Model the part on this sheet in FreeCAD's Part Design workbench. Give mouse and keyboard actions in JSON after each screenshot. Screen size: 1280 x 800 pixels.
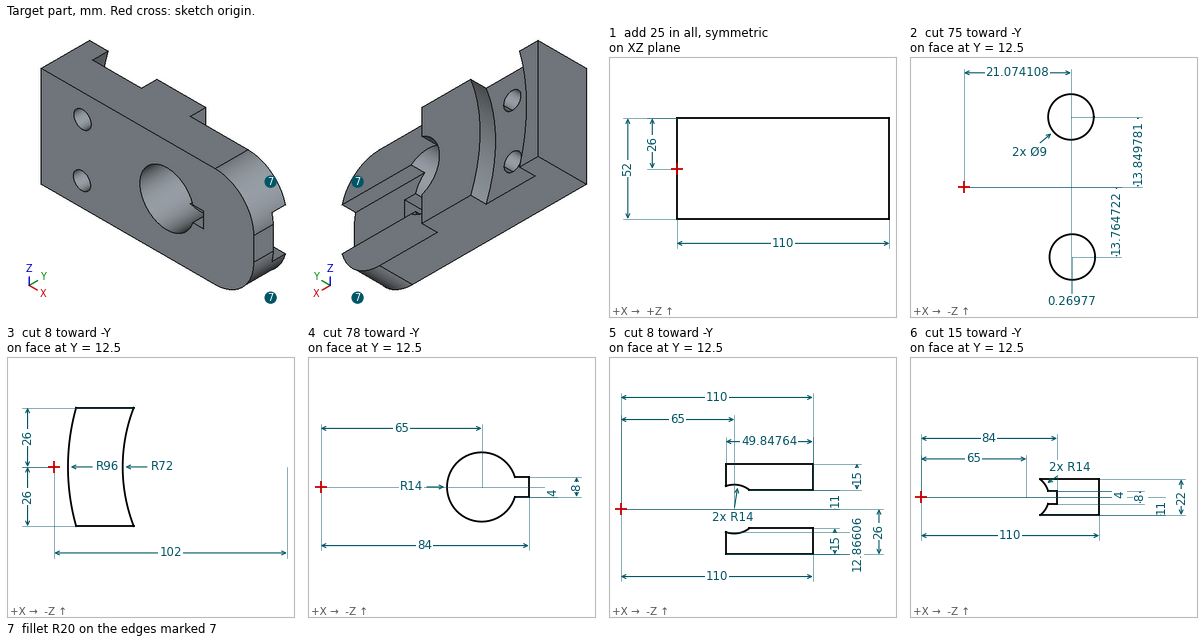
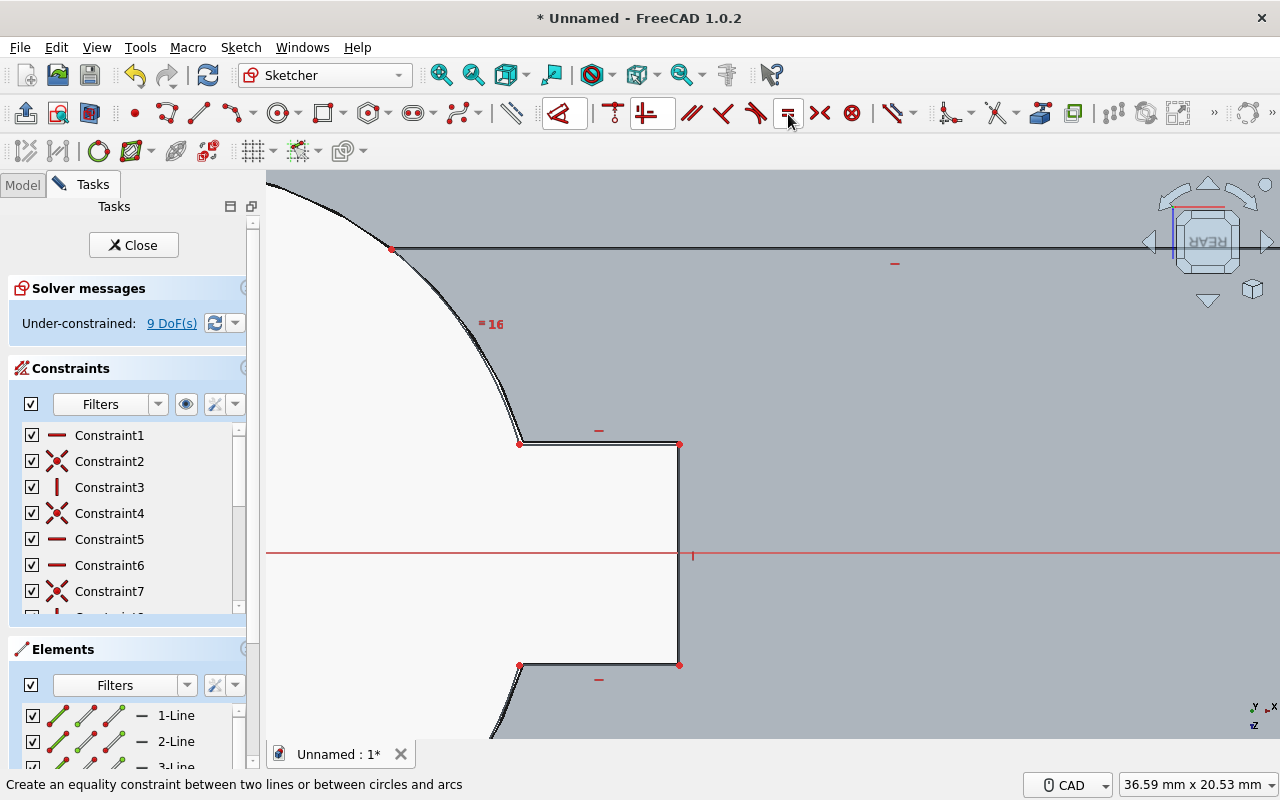
{"action": "scroll", "coordinate": [472, 334], "scroll_direction": "down", "scroll_amount": 3}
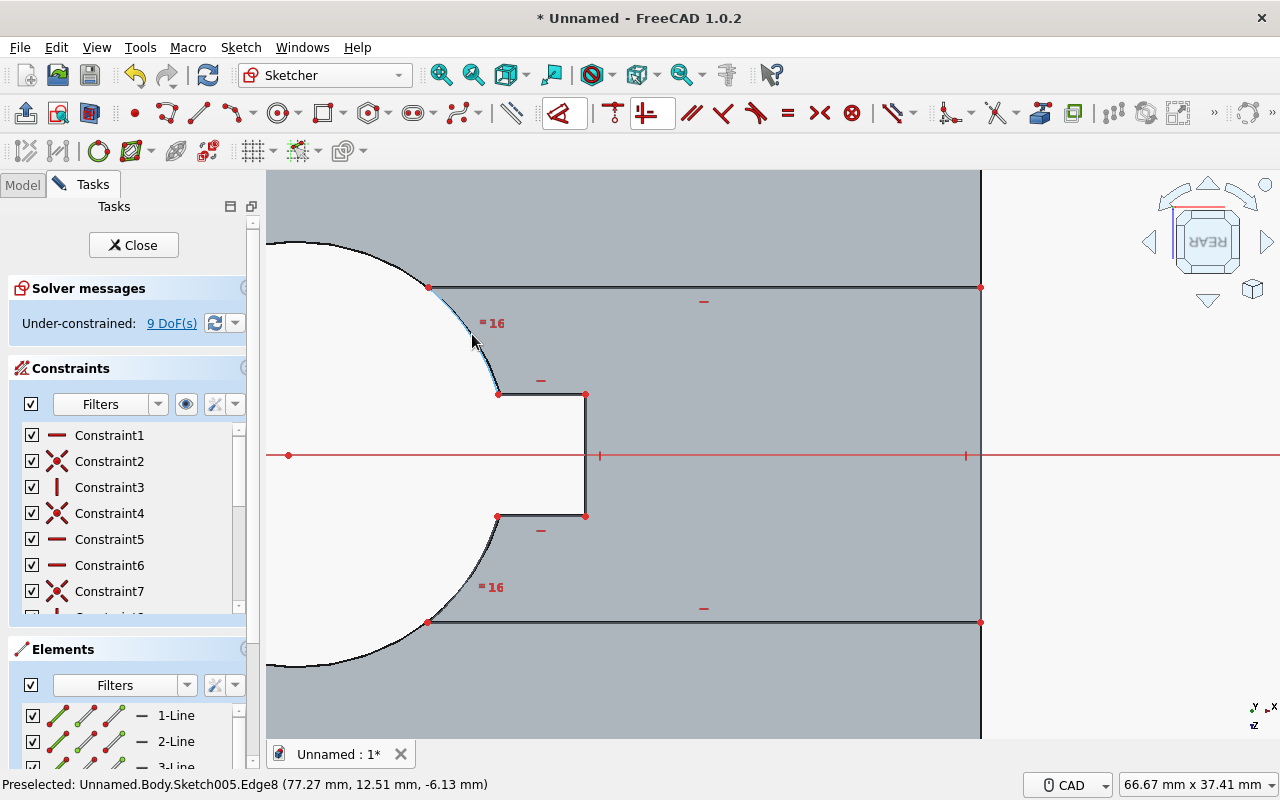
{"action": "scroll", "coordinate": [1020, 455], "scroll_direction": "down", "scroll_amount": 1}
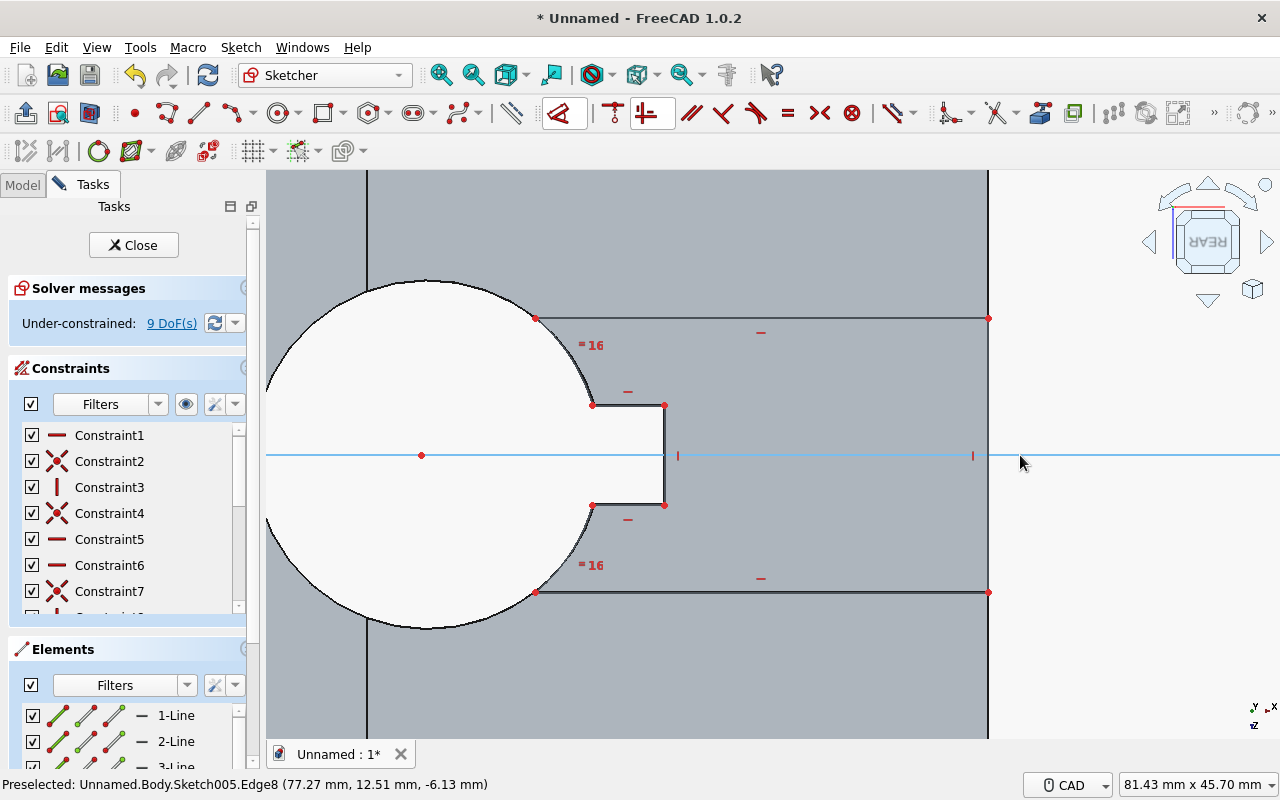
{"action": "left_click", "coordinate": [421, 455]}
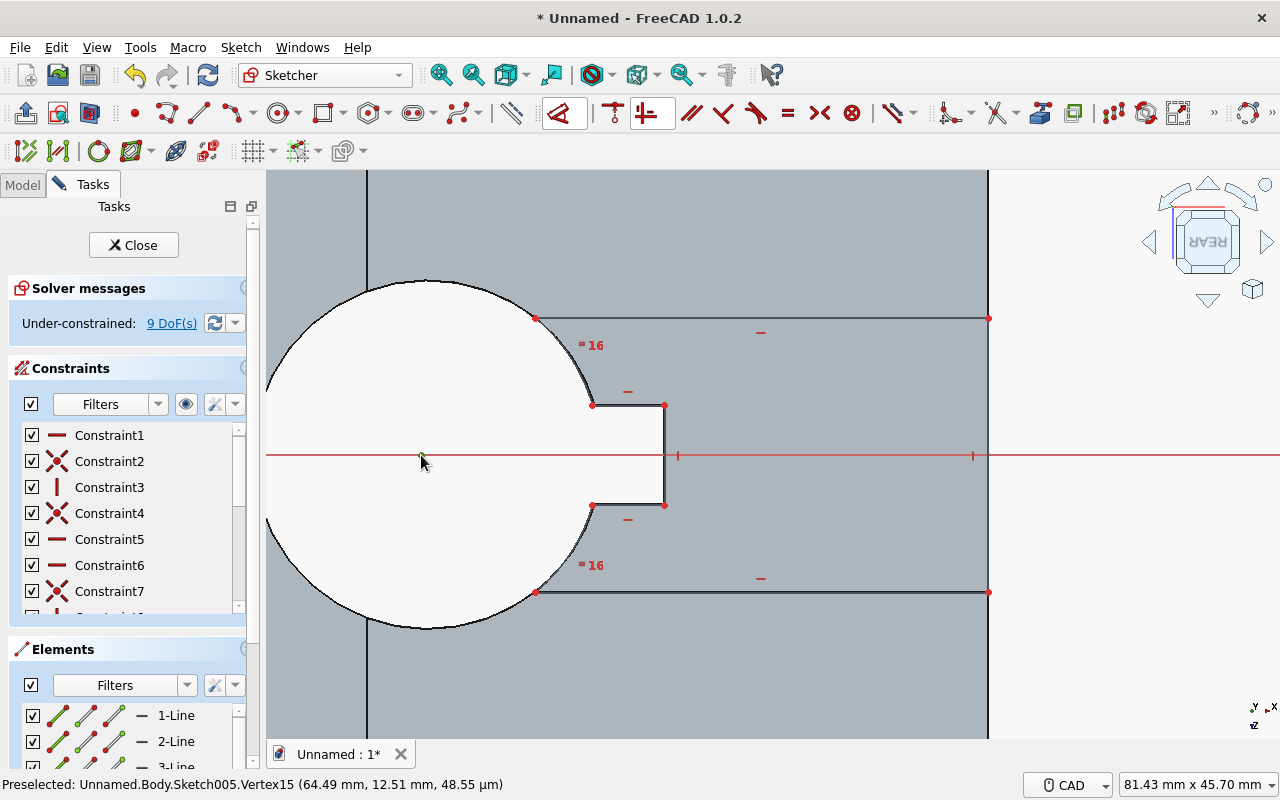
{"action": "left_click", "coordinate": [353, 455]}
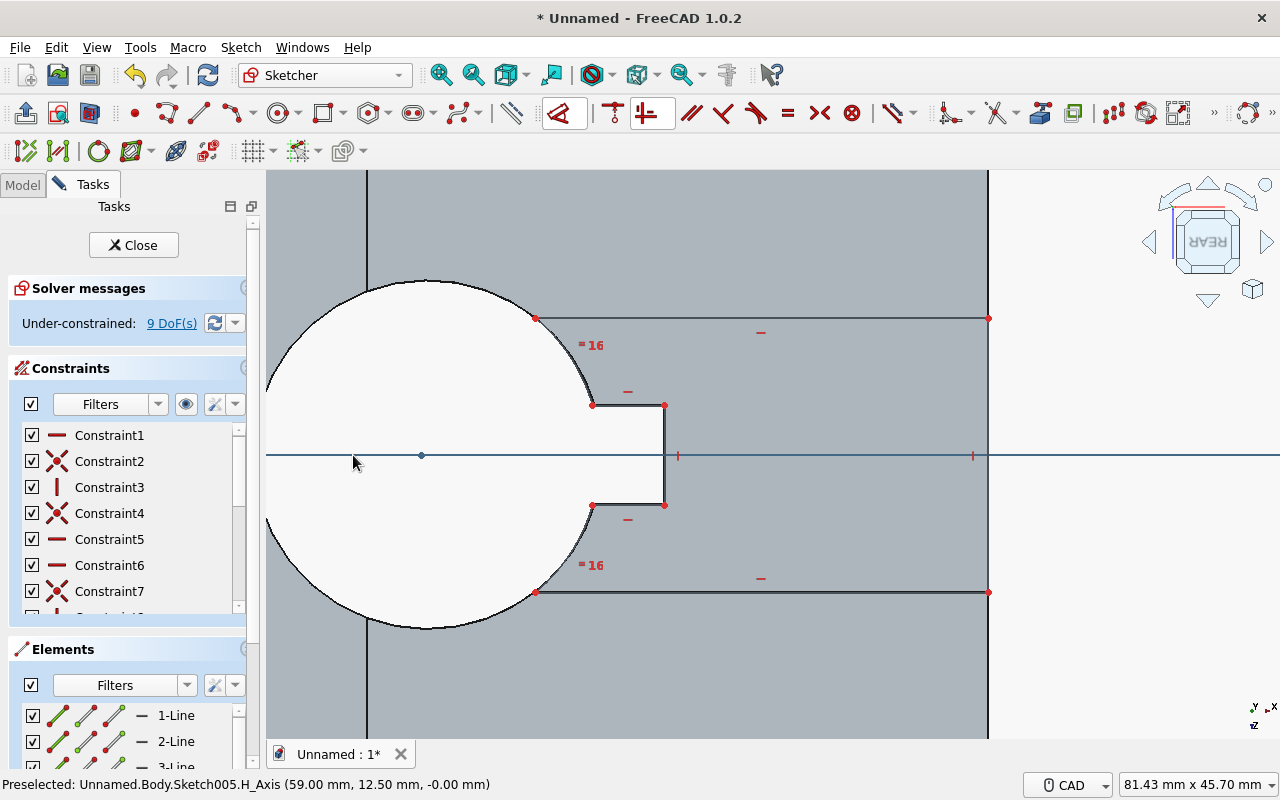
{"action": "left_click", "coordinate": [614, 114]}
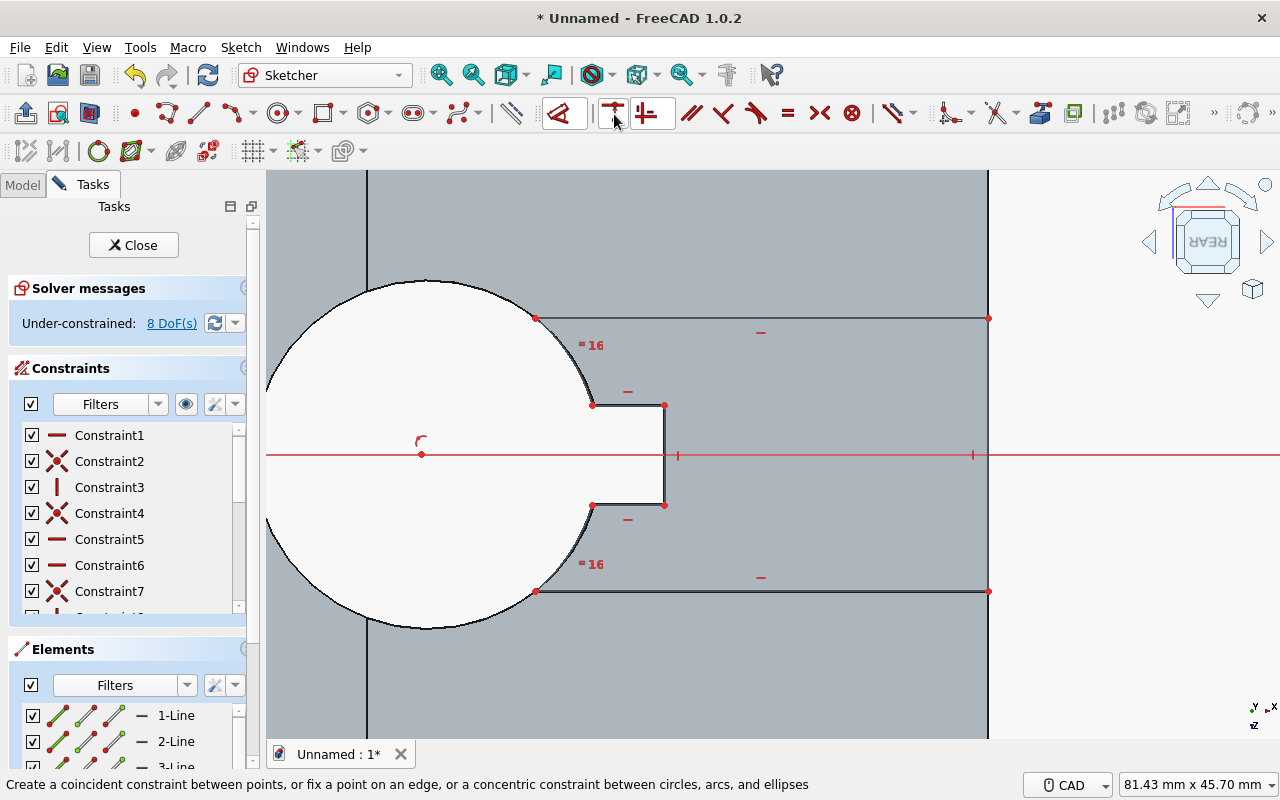
{"action": "left_click", "coordinate": [558, 569]}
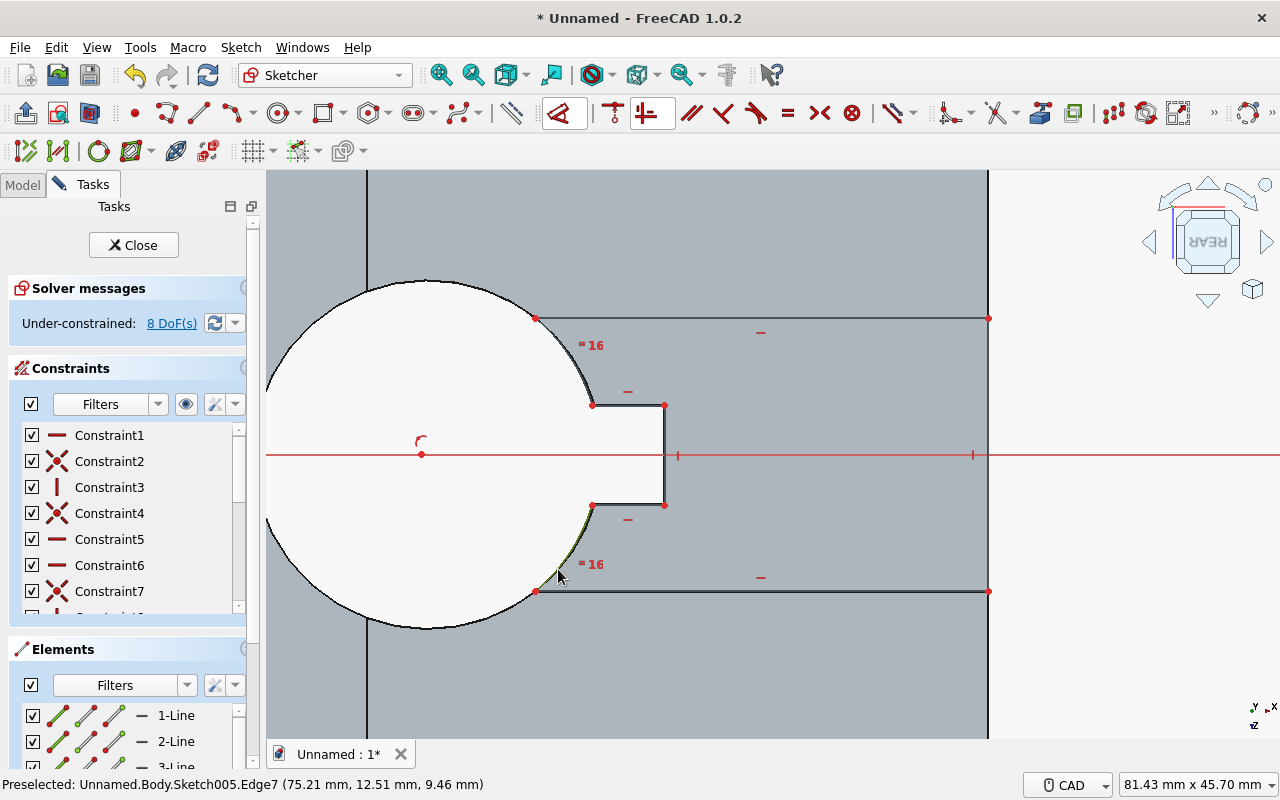
{"action": "left_click", "coordinate": [582, 114]}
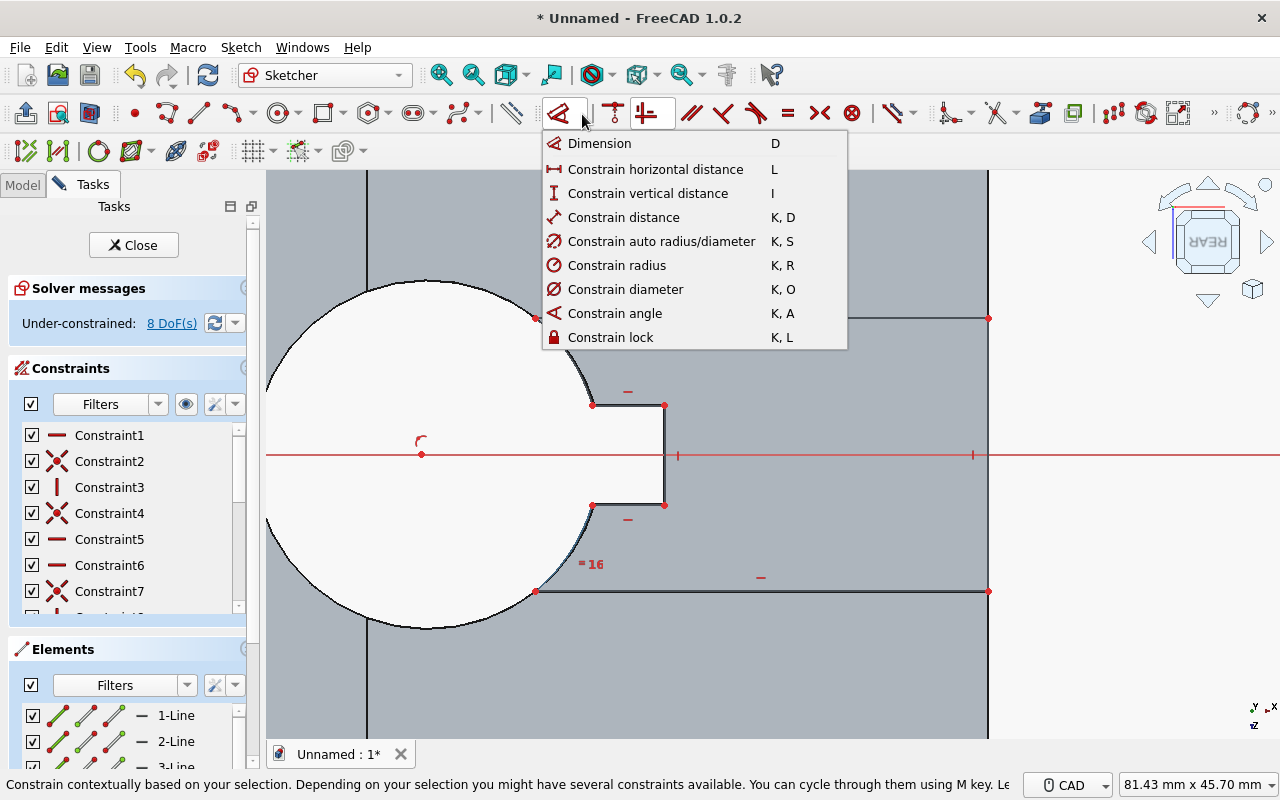
{"action": "left_click", "coordinate": [695, 265]}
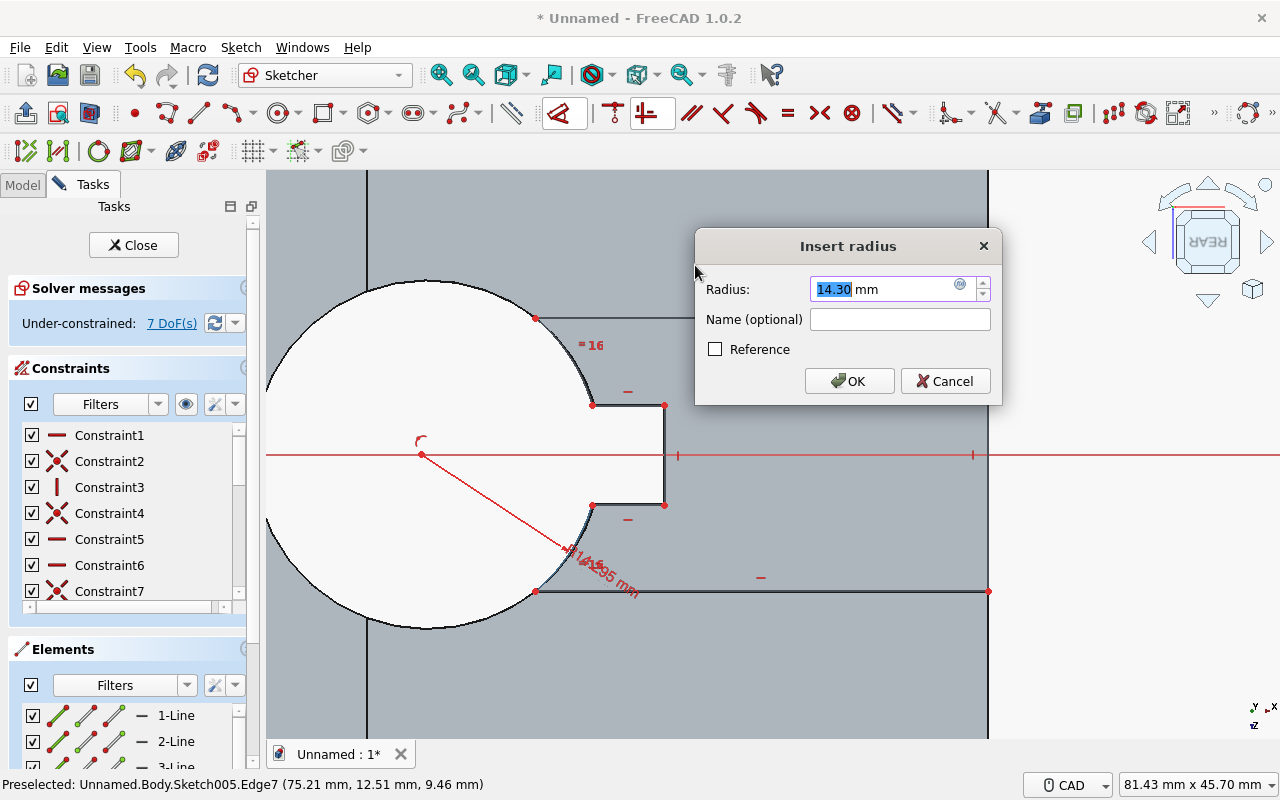
{"action": "type", "text": "14"}
{"action": "key", "text": "Return"}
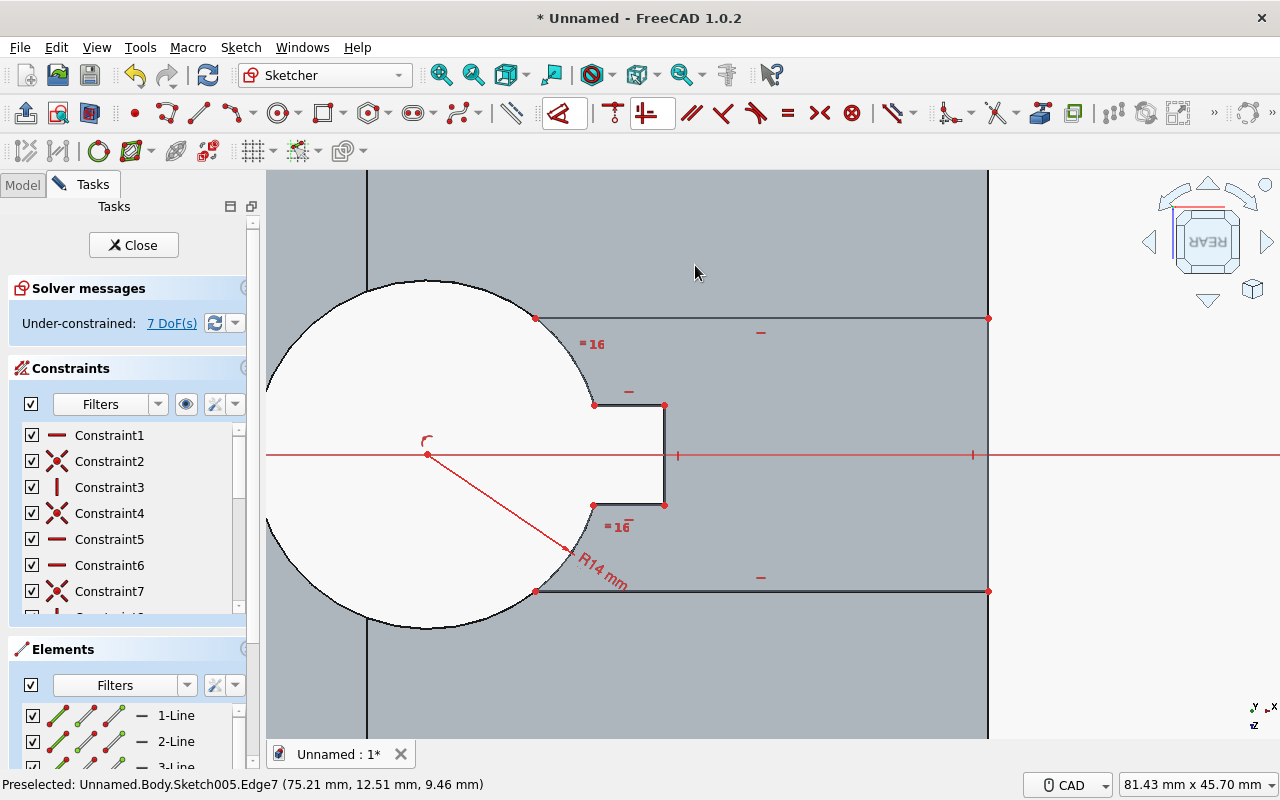
{"action": "left_click", "coordinate": [665, 436]}